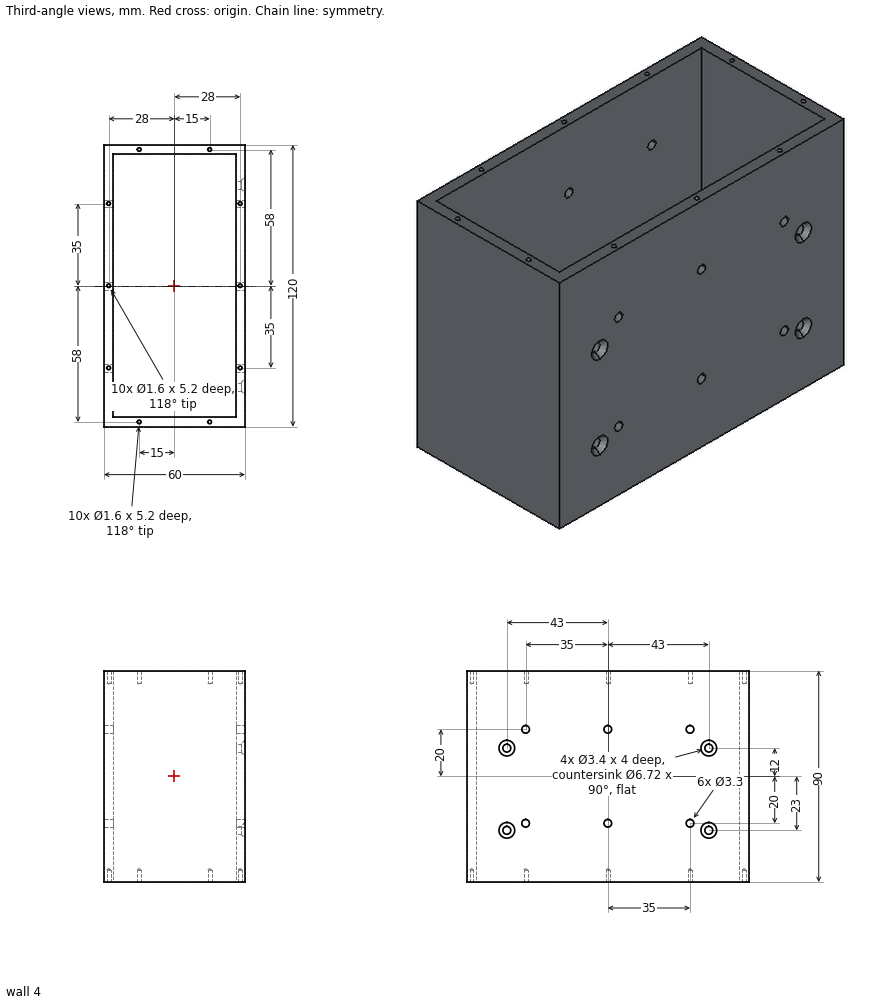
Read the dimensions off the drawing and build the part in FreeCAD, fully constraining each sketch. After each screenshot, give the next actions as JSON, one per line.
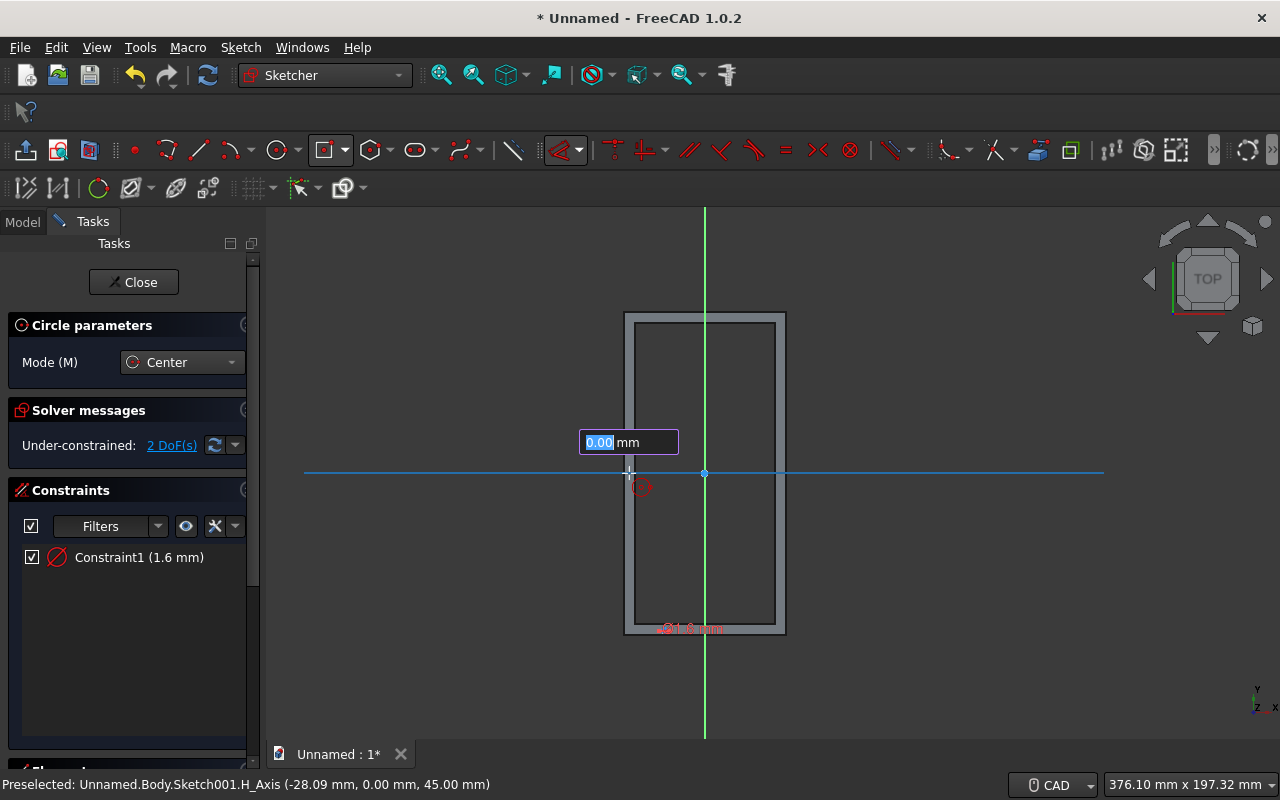
{"action": "scroll", "coordinate": [630, 471], "scroll_direction": "up", "scroll_amount": 11}
{"action": "mouse_move", "coordinate": [627, 471]}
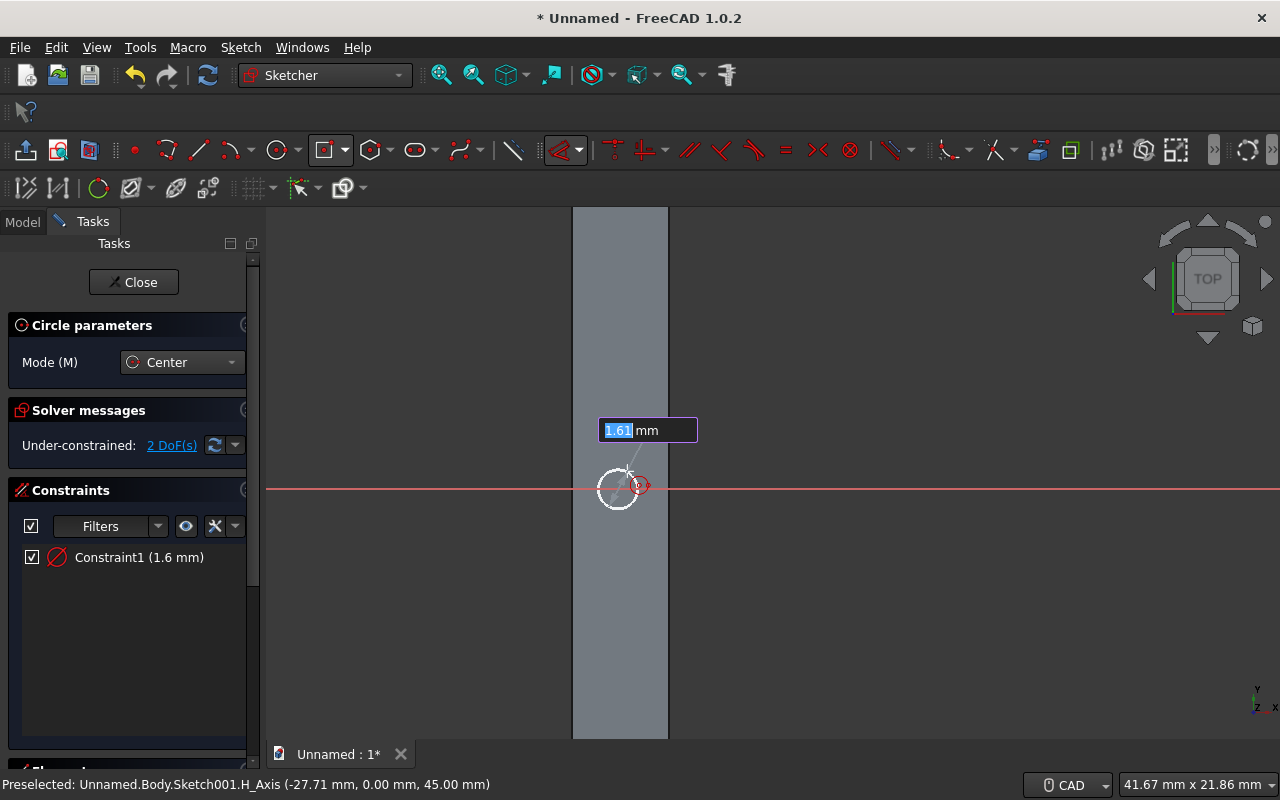
{"action": "type", "text": "1.6"}
{"action": "key", "text": "Return"}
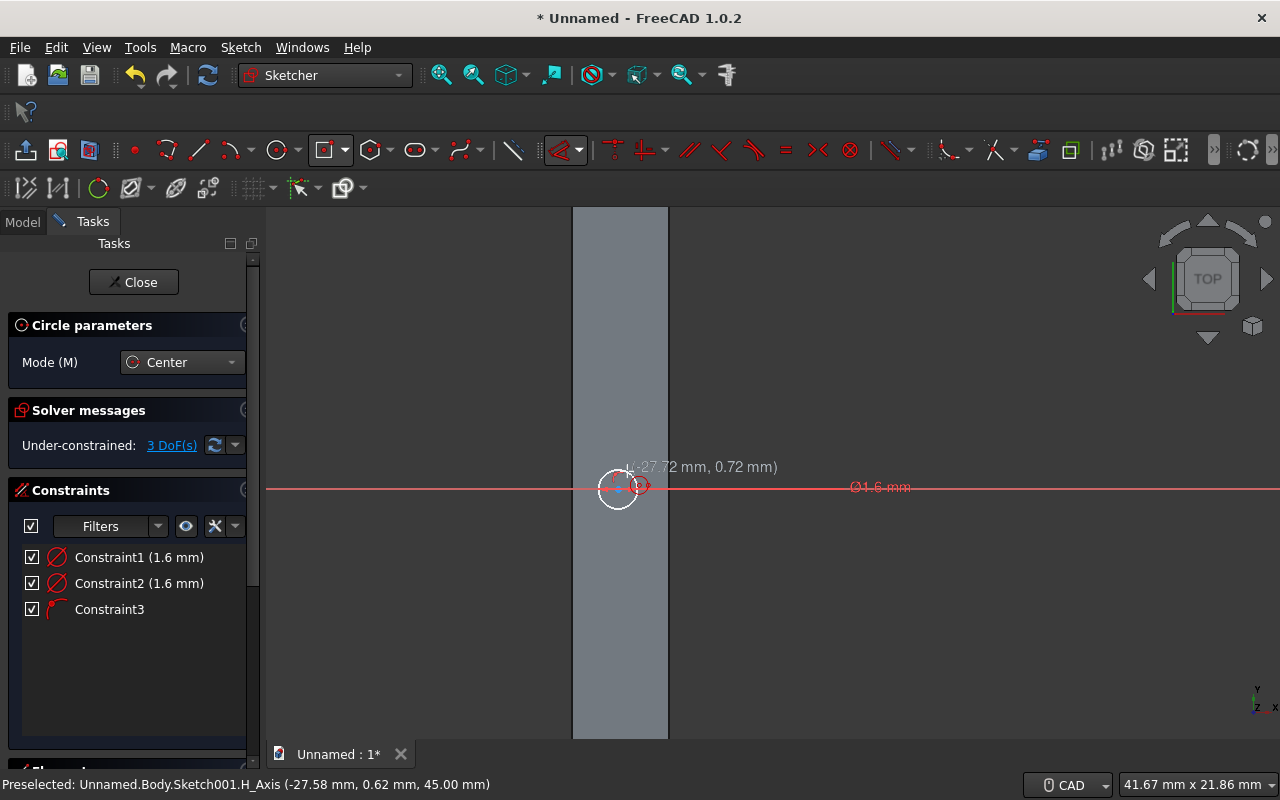
{"action": "scroll", "coordinate": [630, 471], "scroll_direction": "down", "scroll_amount": 11}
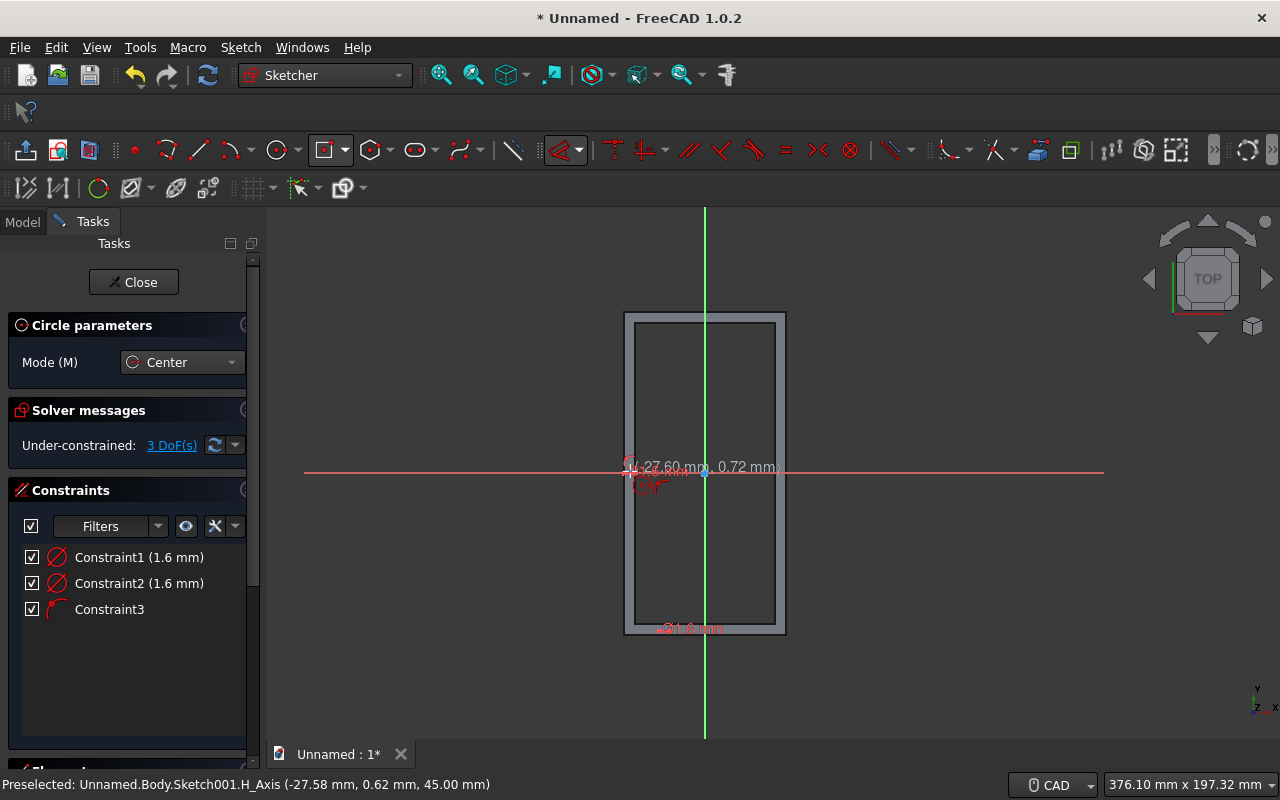
{"action": "scroll", "coordinate": [780, 473], "scroll_direction": "up", "scroll_amount": 12}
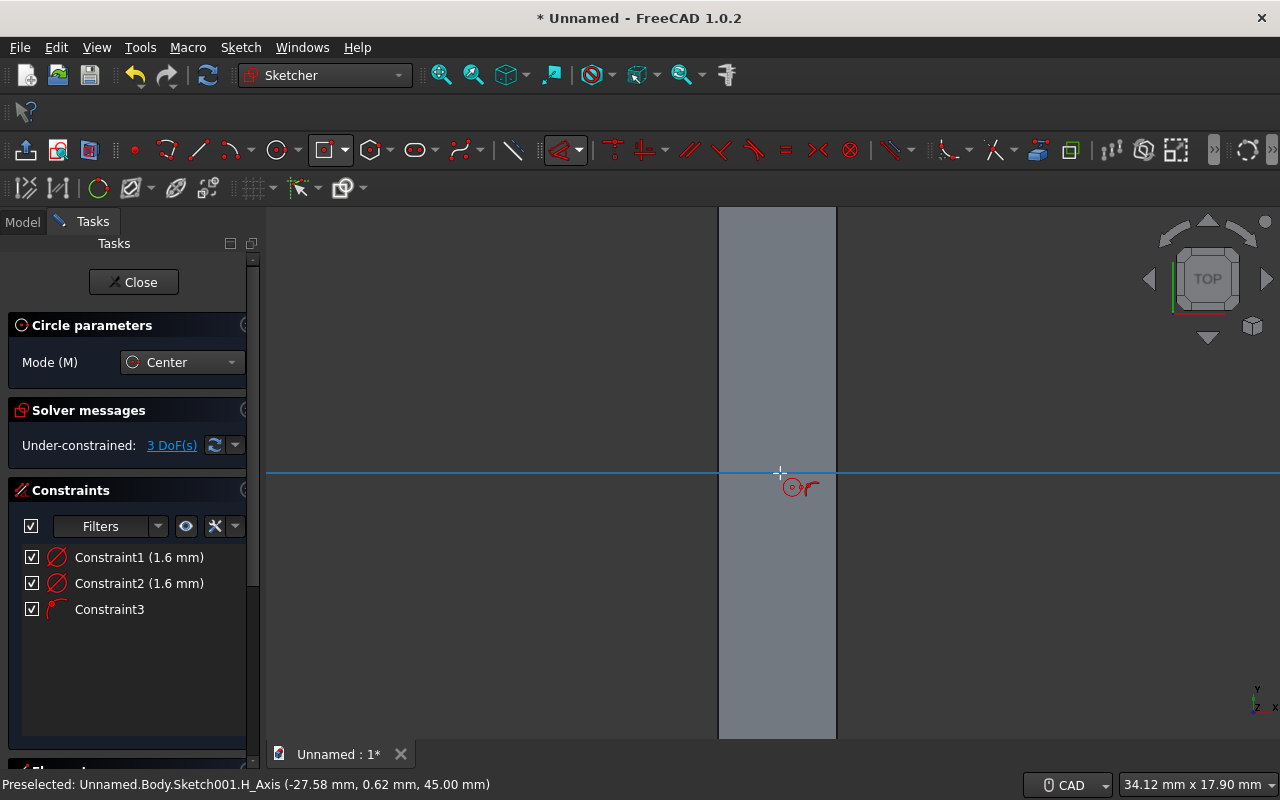
{"action": "scroll", "coordinate": [780, 473], "scroll_direction": "down", "scroll_amount": 12}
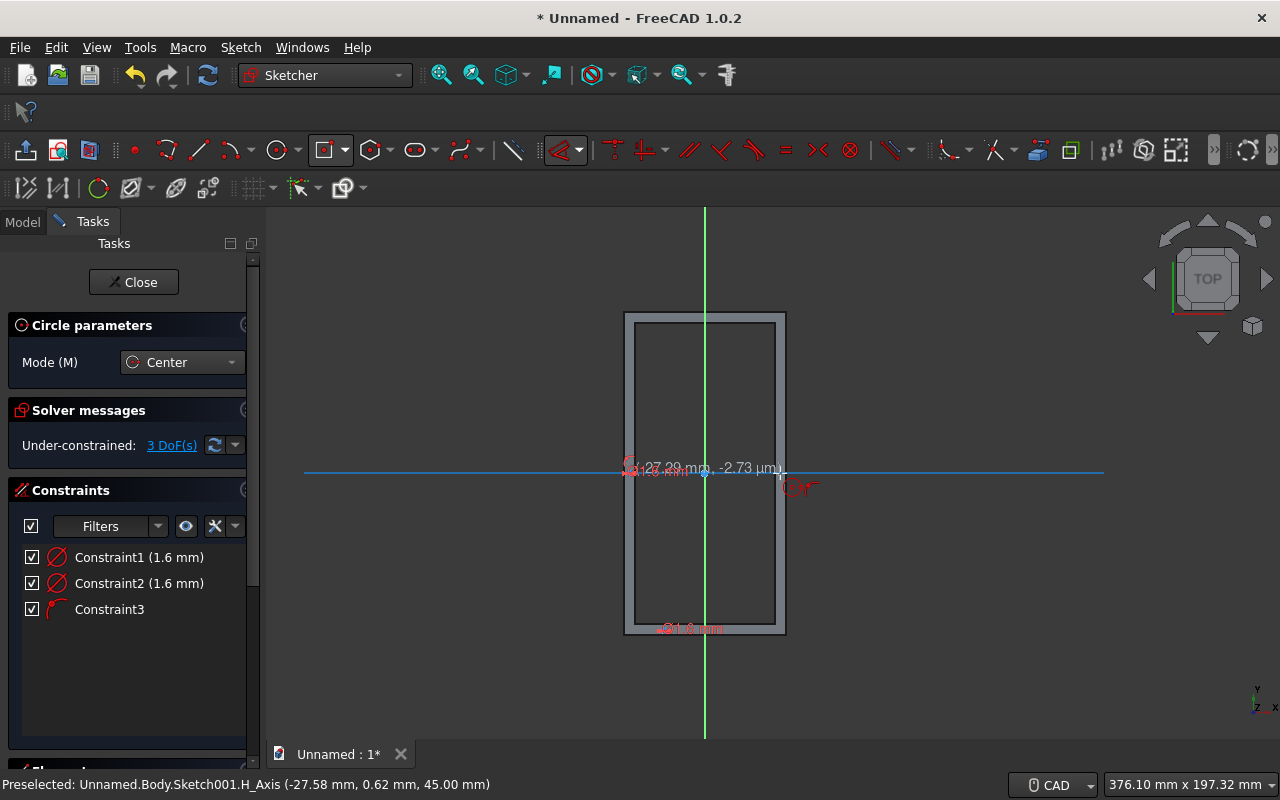
{"action": "left_click", "coordinate": [780, 473]}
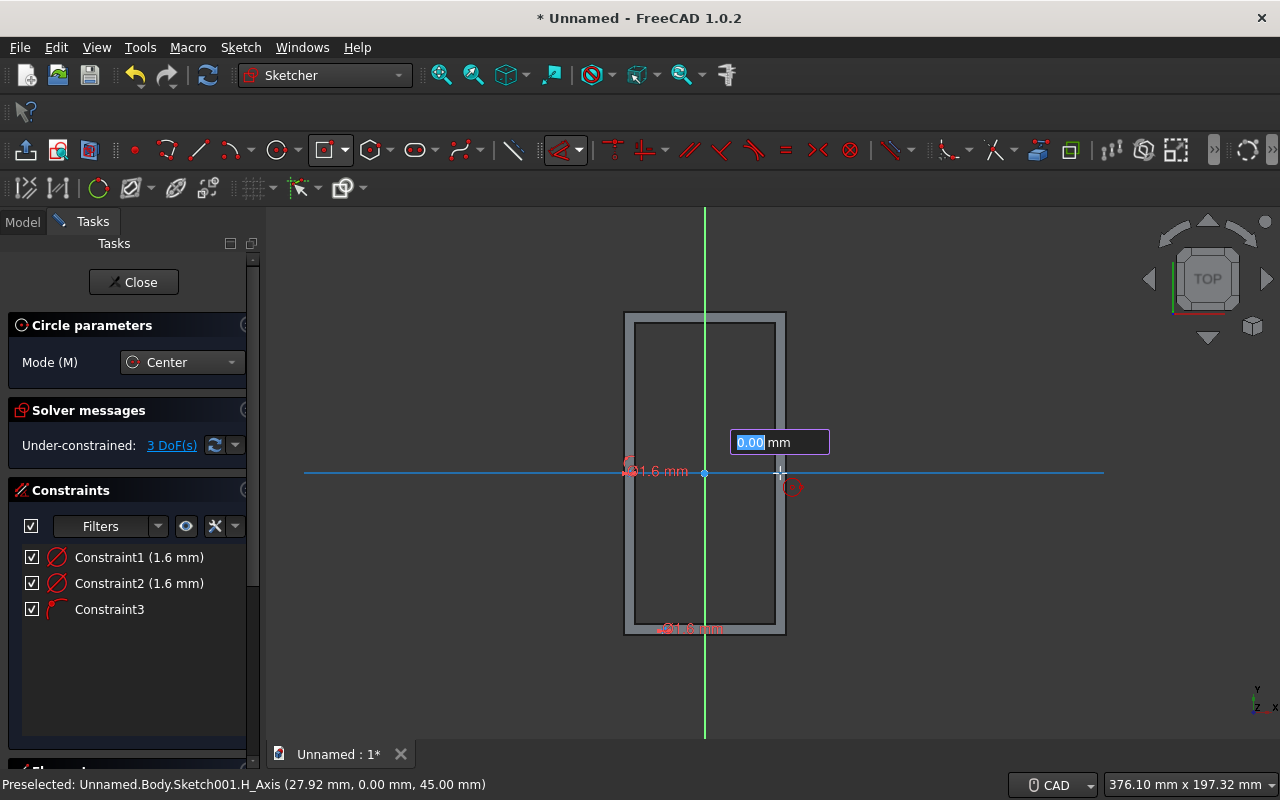
{"action": "scroll", "coordinate": [779, 476], "scroll_direction": "up", "scroll_amount": 11}
{"action": "mouse_move", "coordinate": [779, 468]}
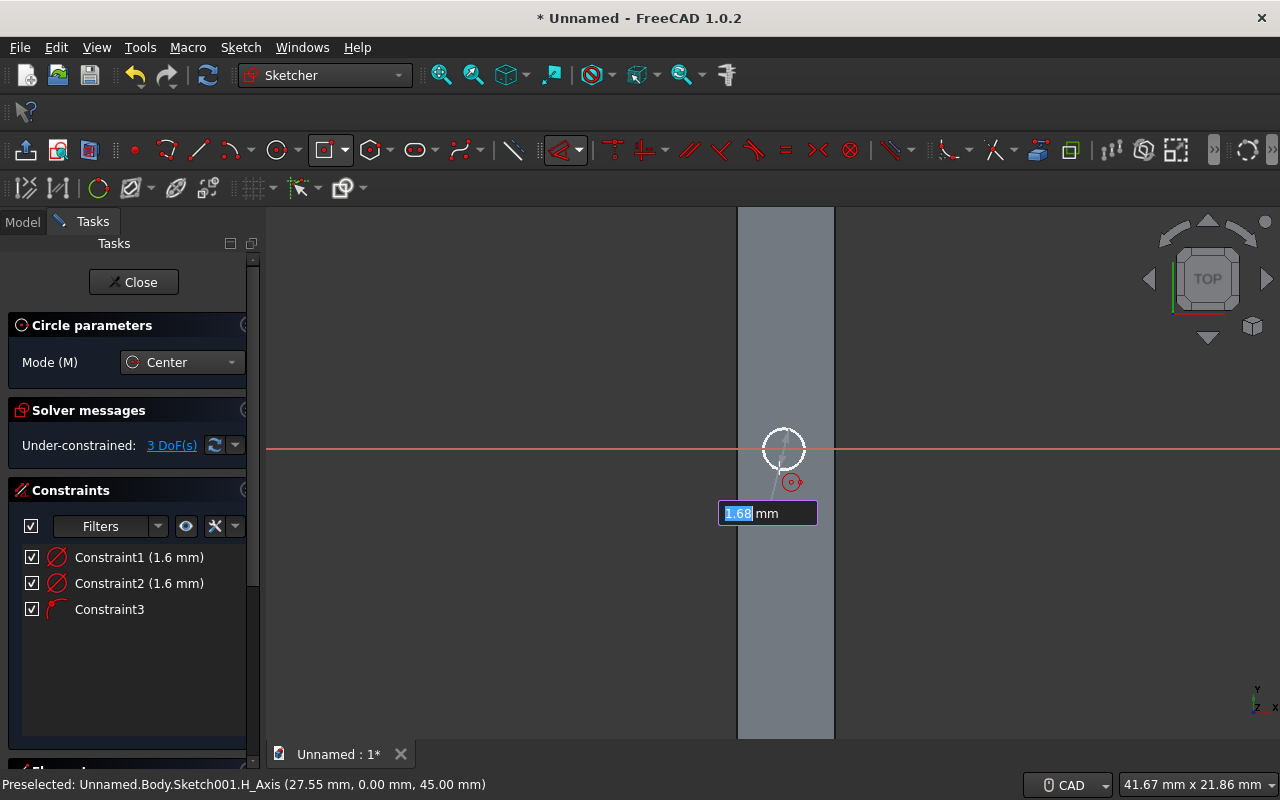
{"action": "type", "text": "1.6"}
{"action": "key", "text": "Return"}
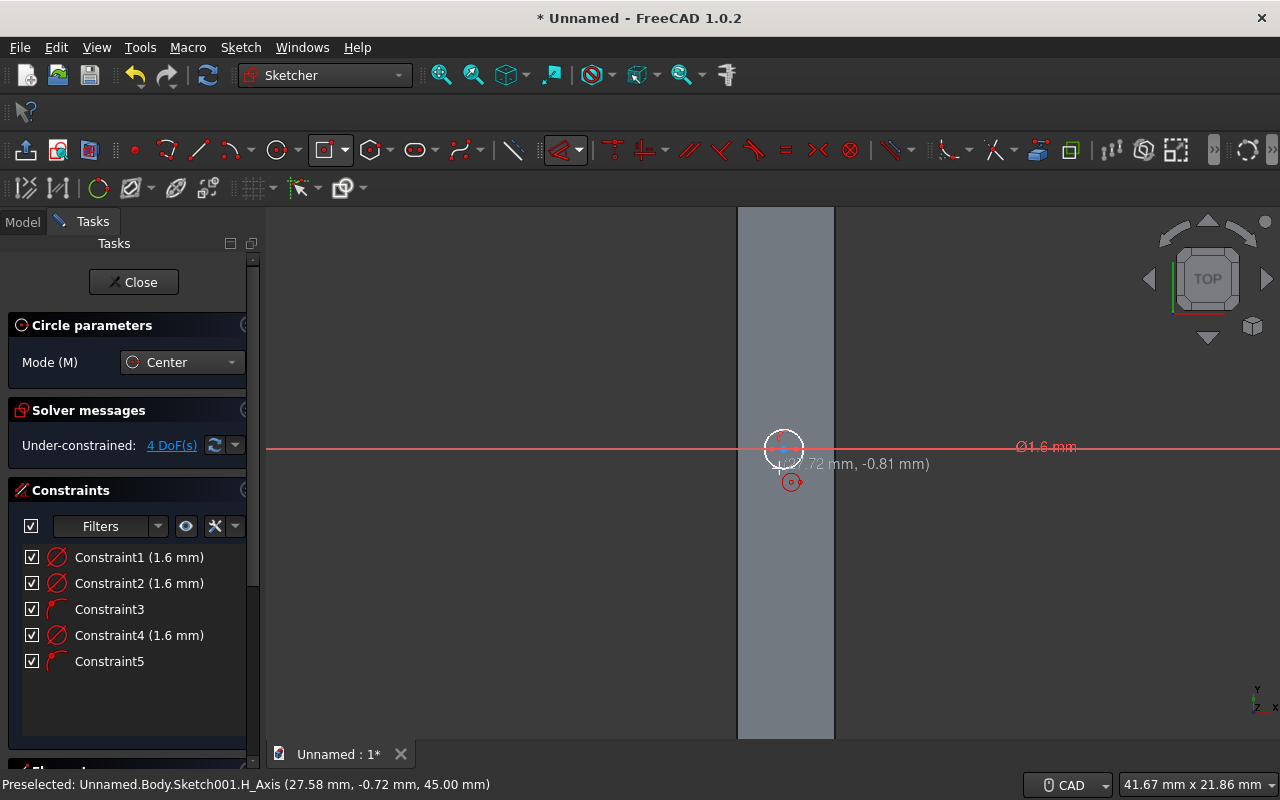
{"action": "scroll", "coordinate": [779, 476], "scroll_direction": "down", "scroll_amount": 11}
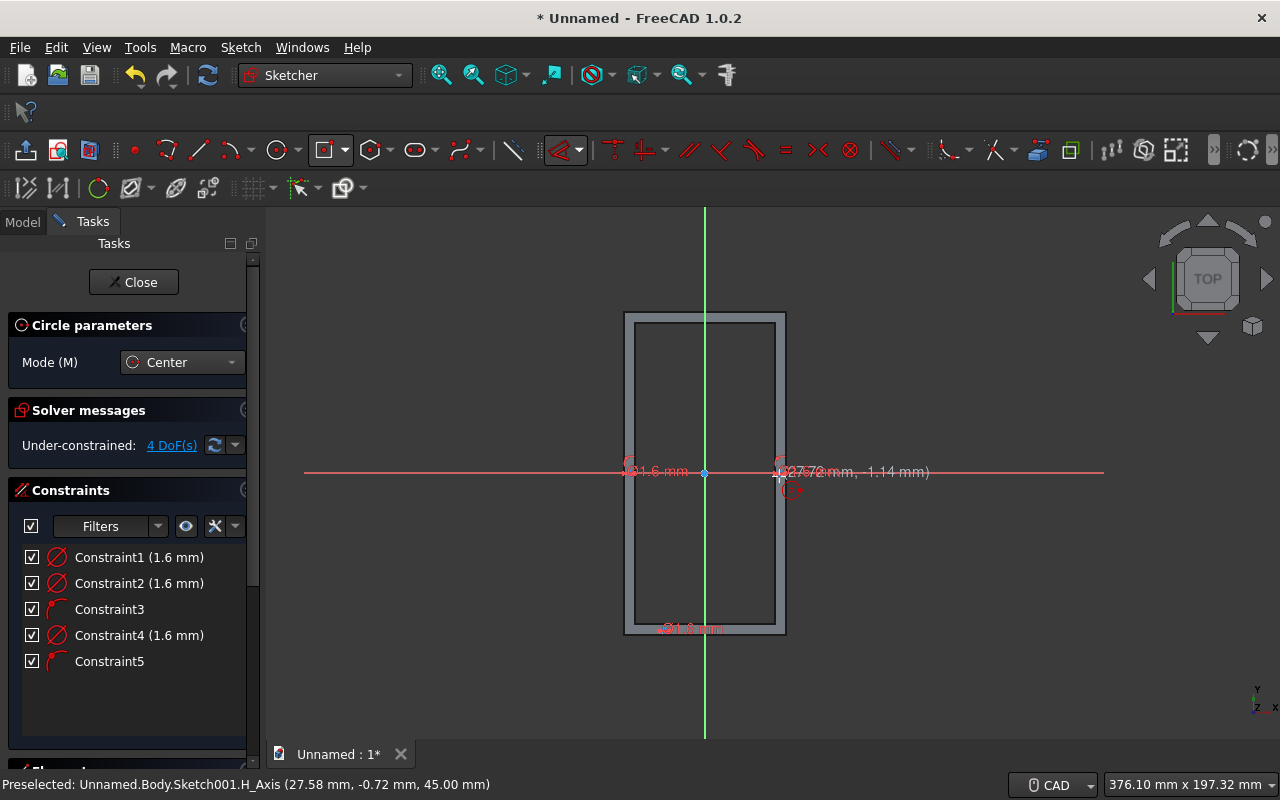
{"action": "scroll", "coordinate": [664, 317], "scroll_direction": "up", "scroll_amount": 12}